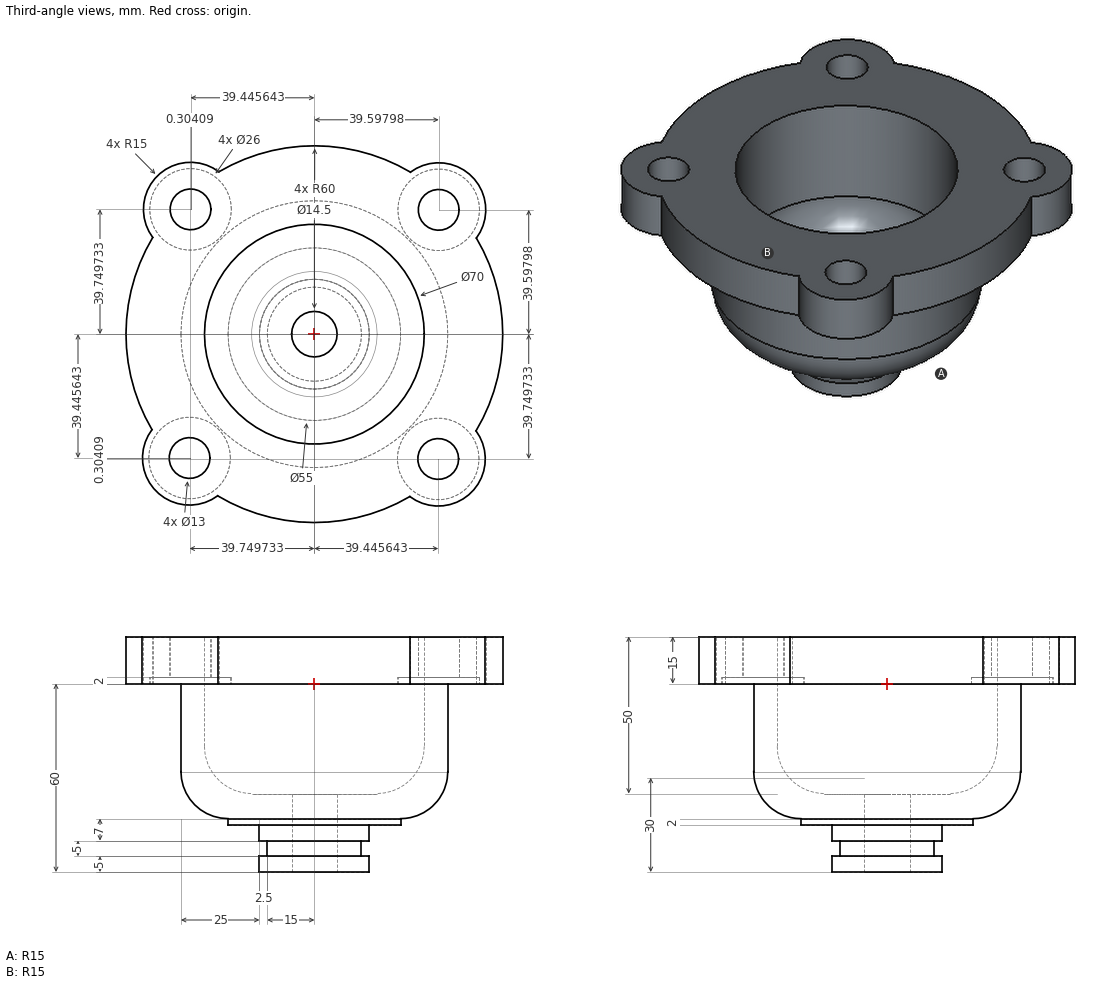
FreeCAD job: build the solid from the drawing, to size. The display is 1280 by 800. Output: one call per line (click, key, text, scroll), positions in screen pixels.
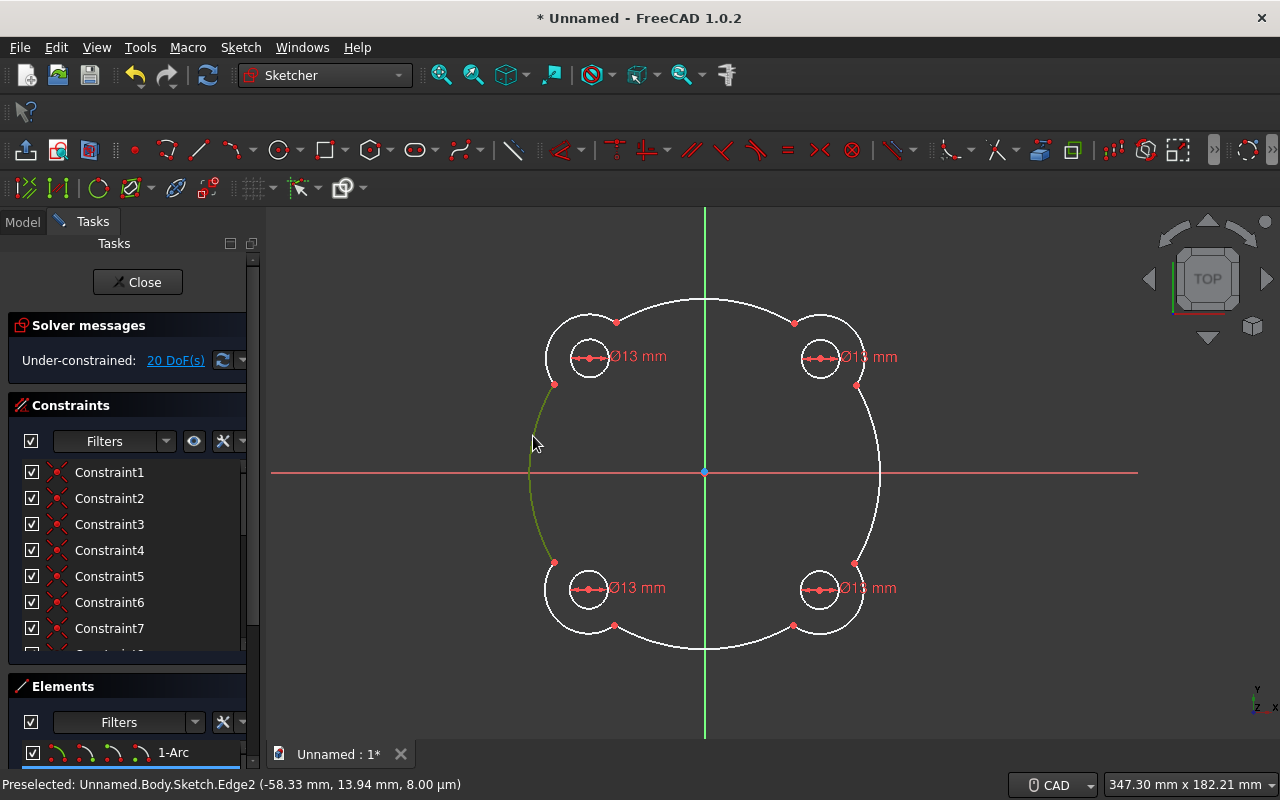
click(742, 303)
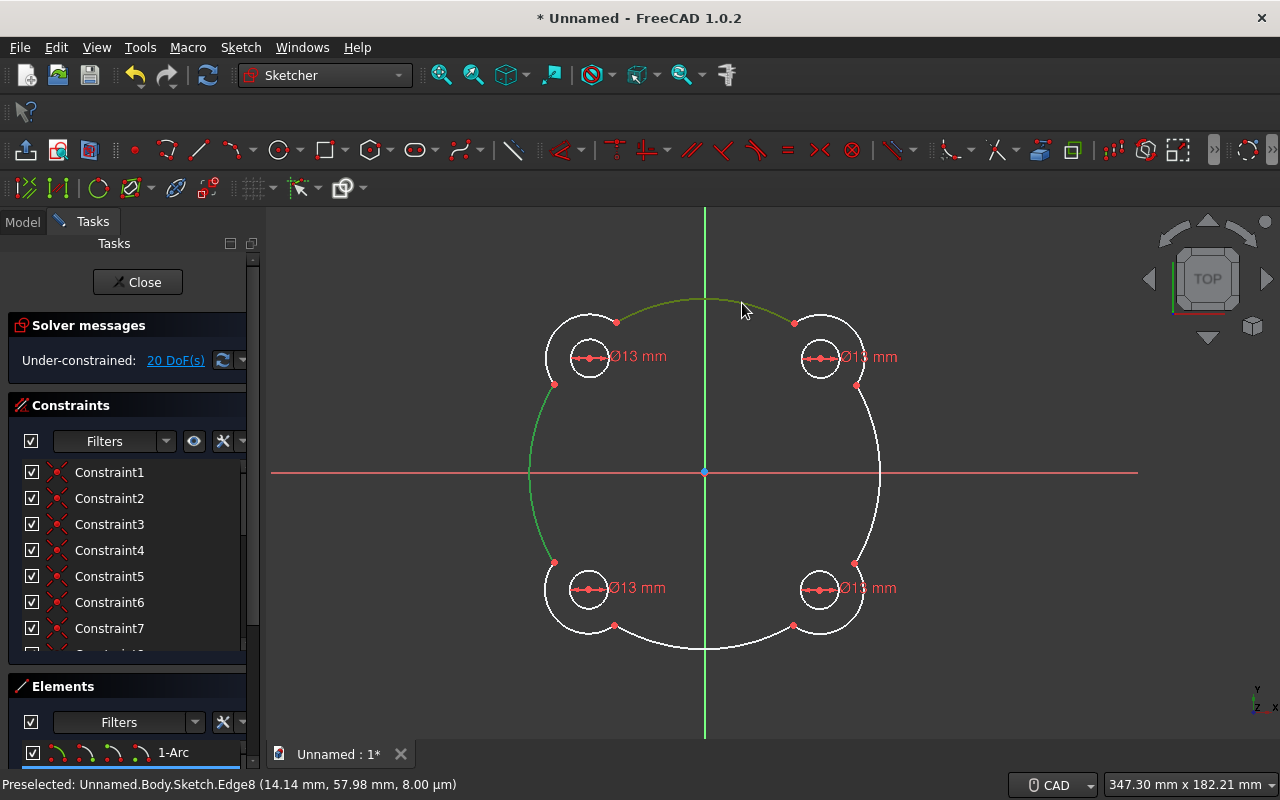
click(616, 150)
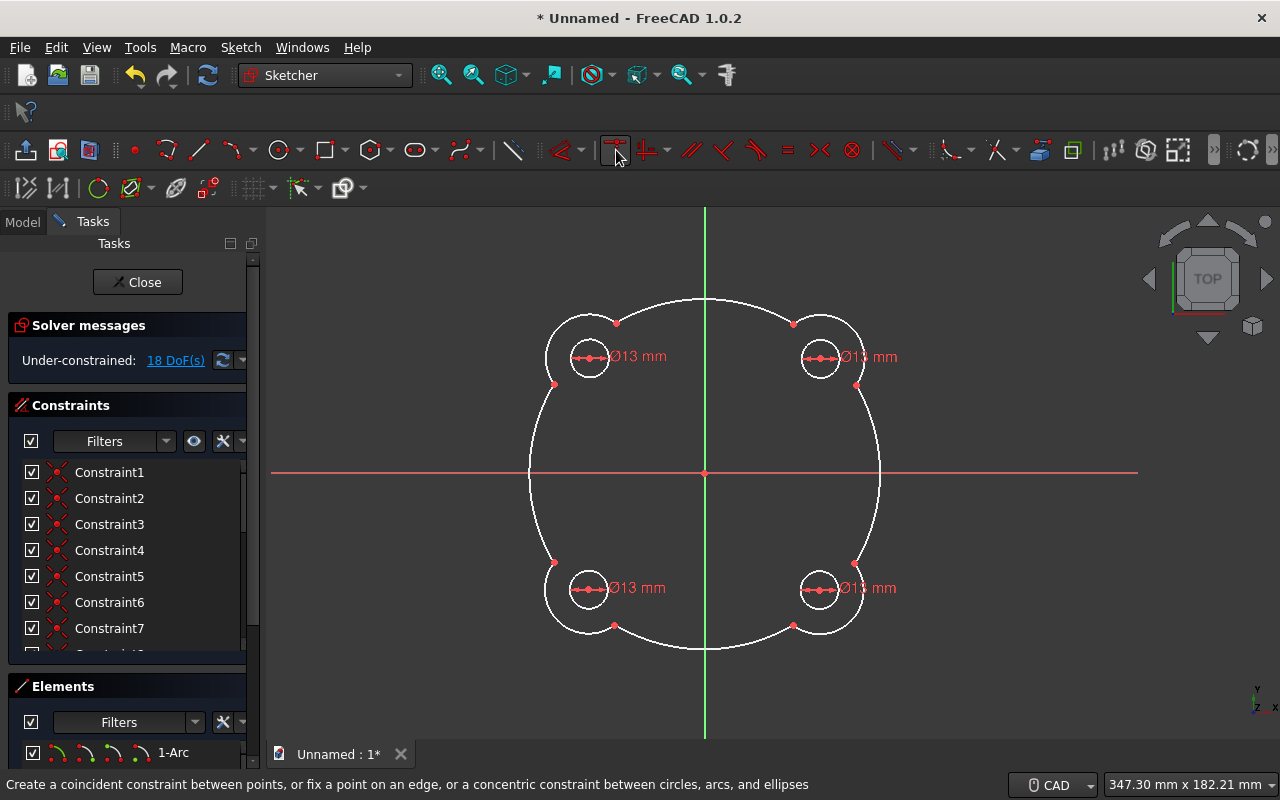
scroll(704, 473, up, 4)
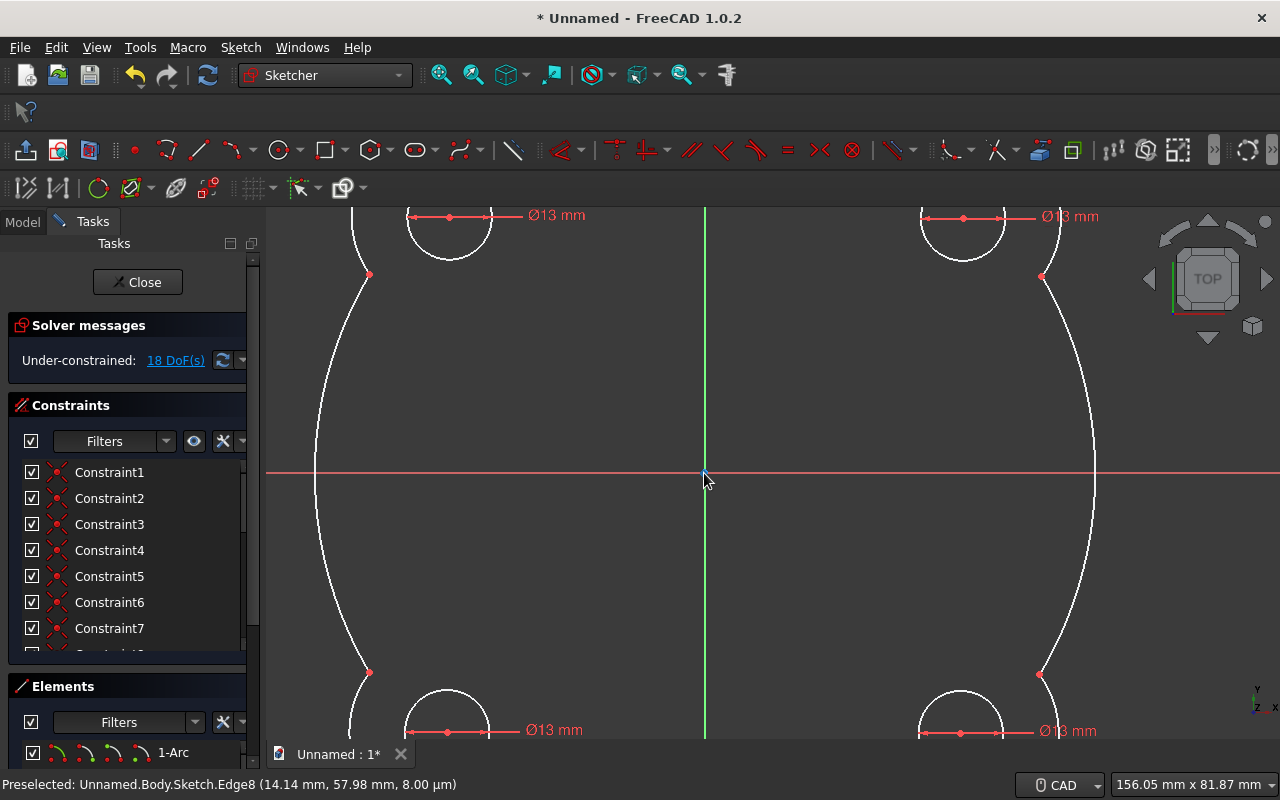
drag(694, 463, 715, 484)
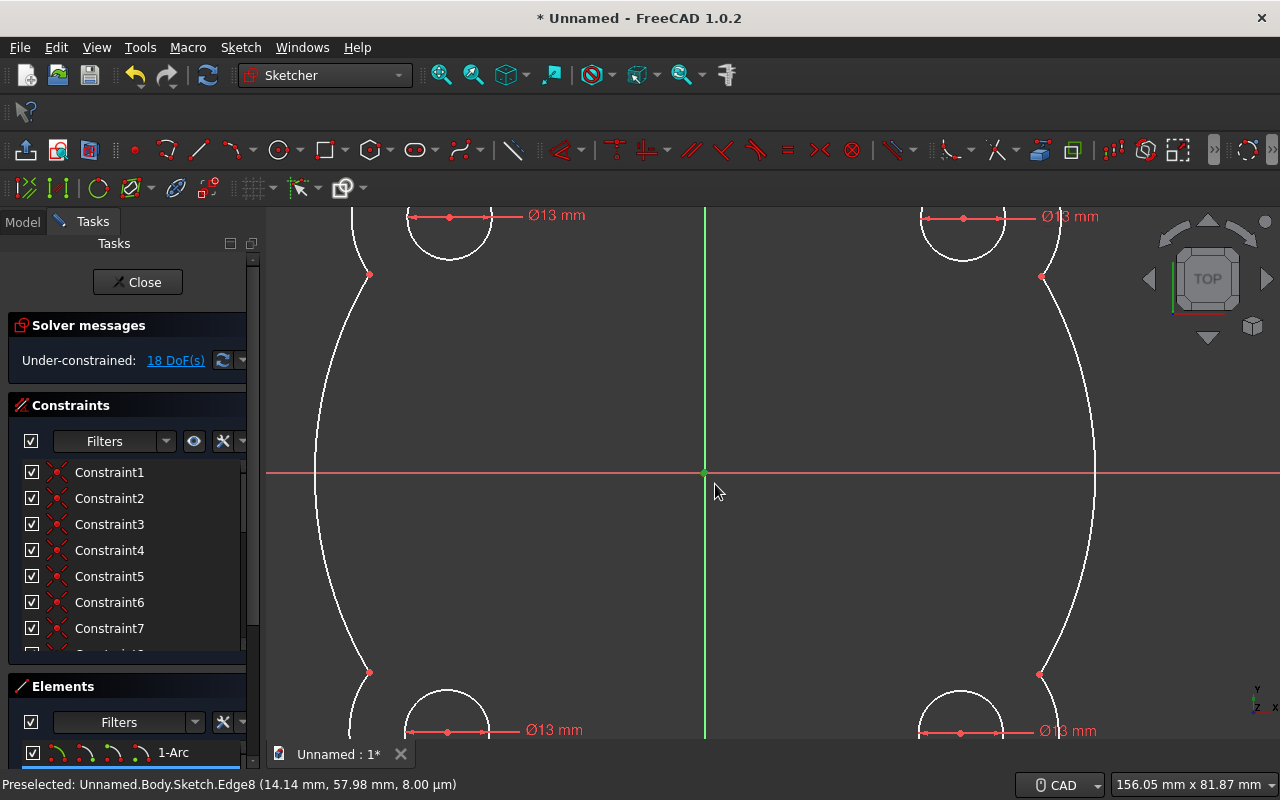
click(616, 150)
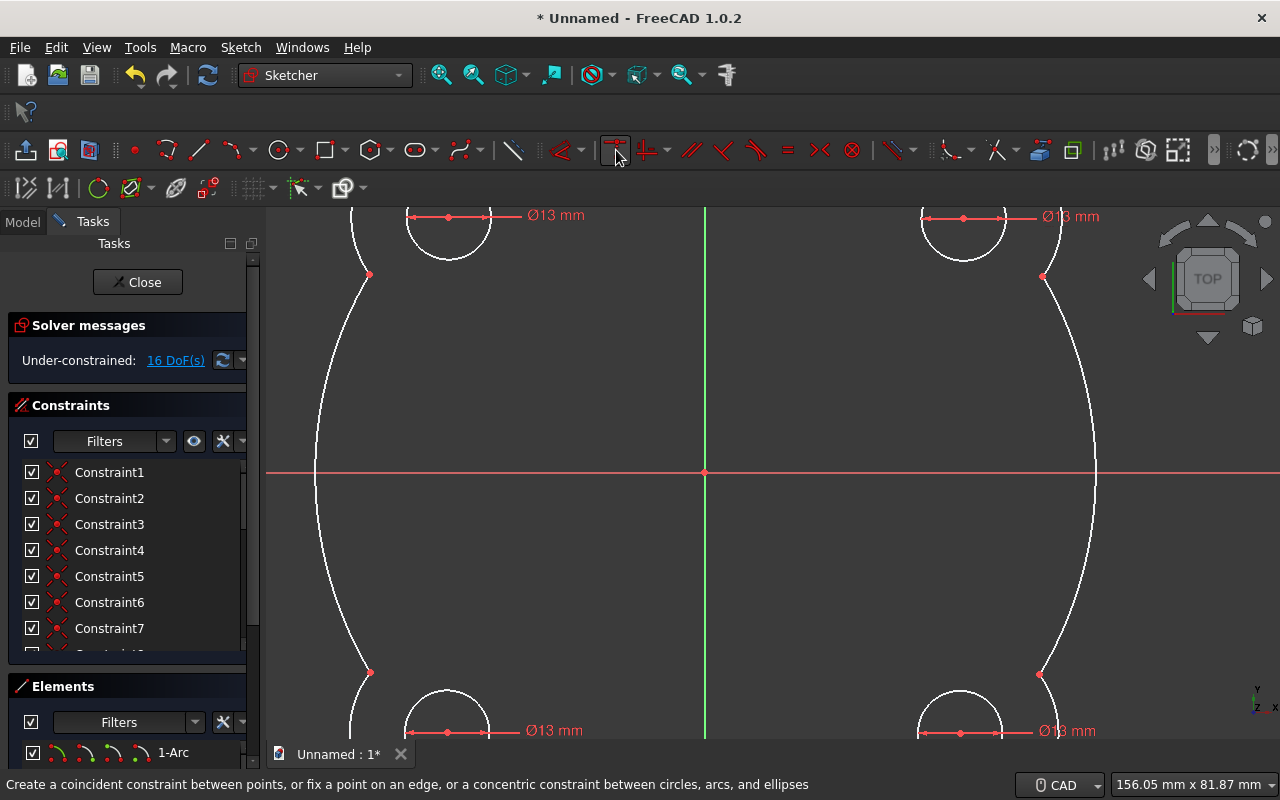
scroll(704, 473, down, 4)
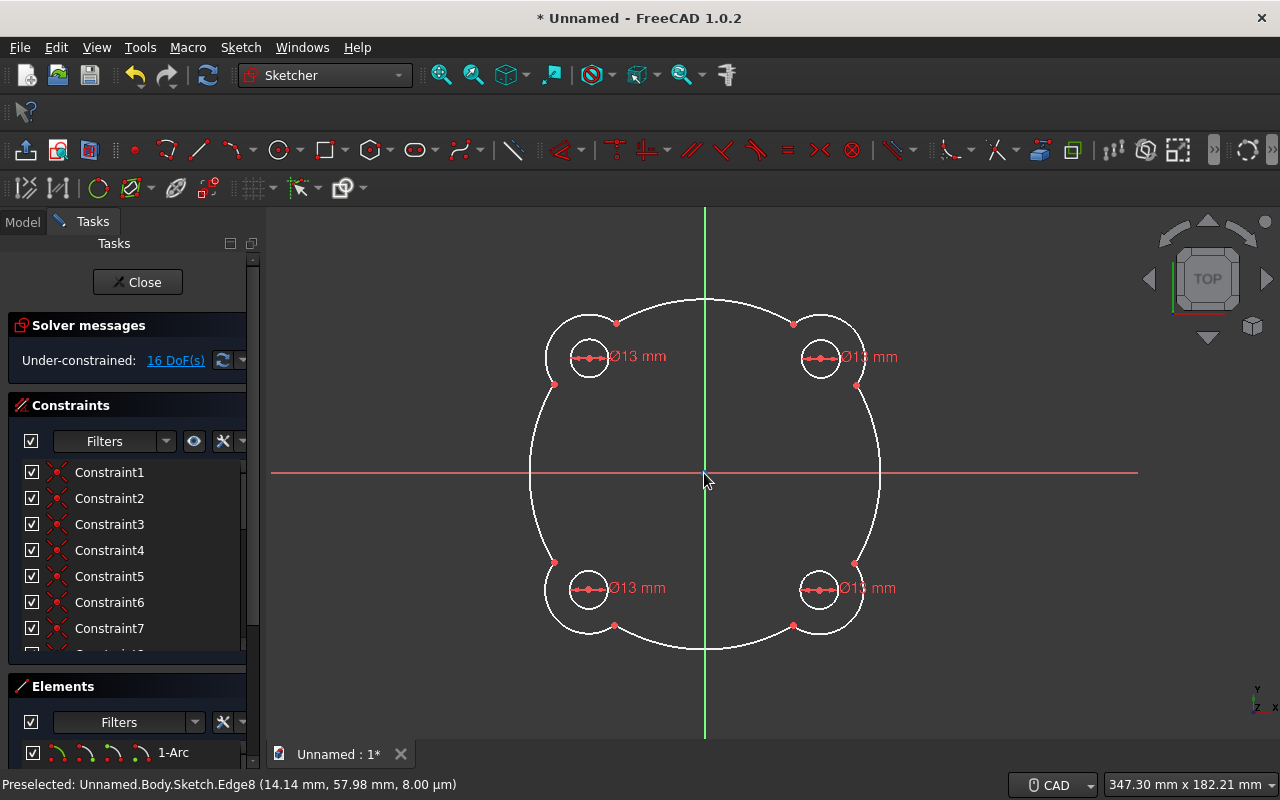
click(581, 316)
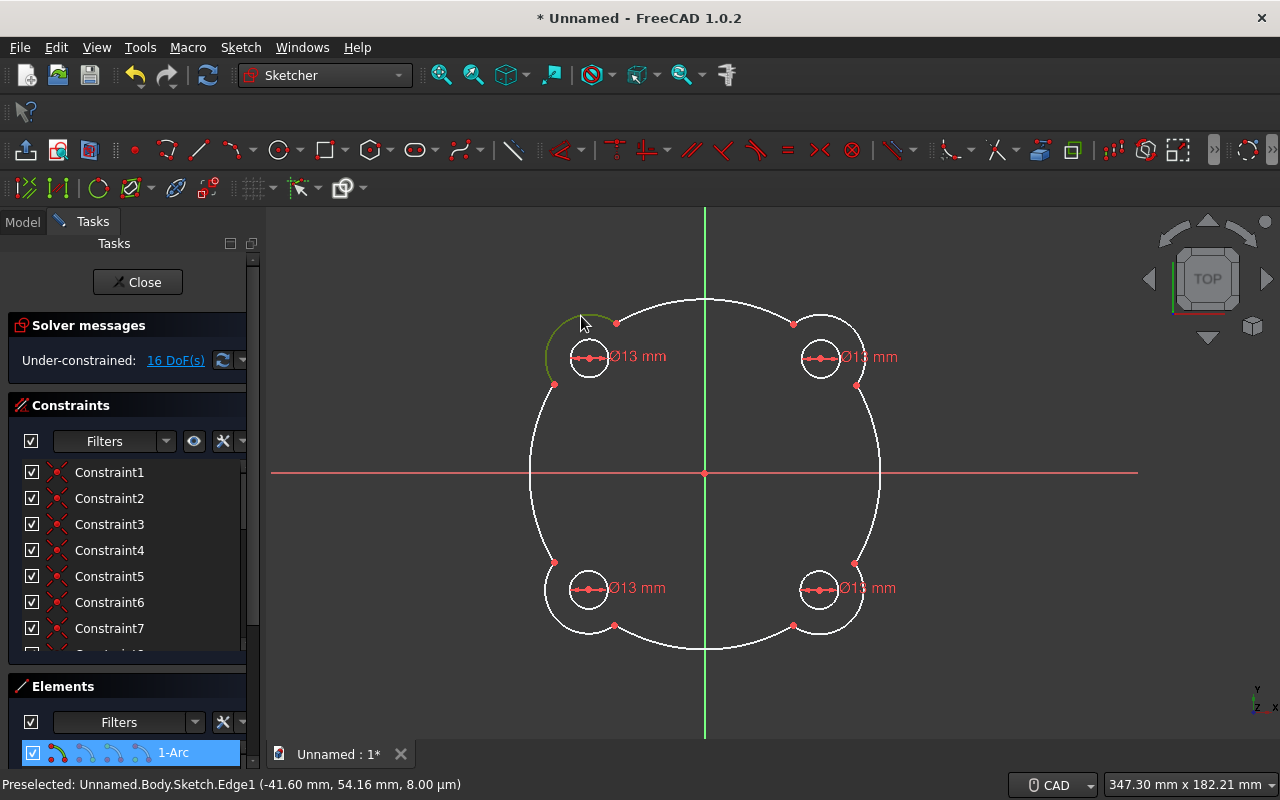
click(546, 599)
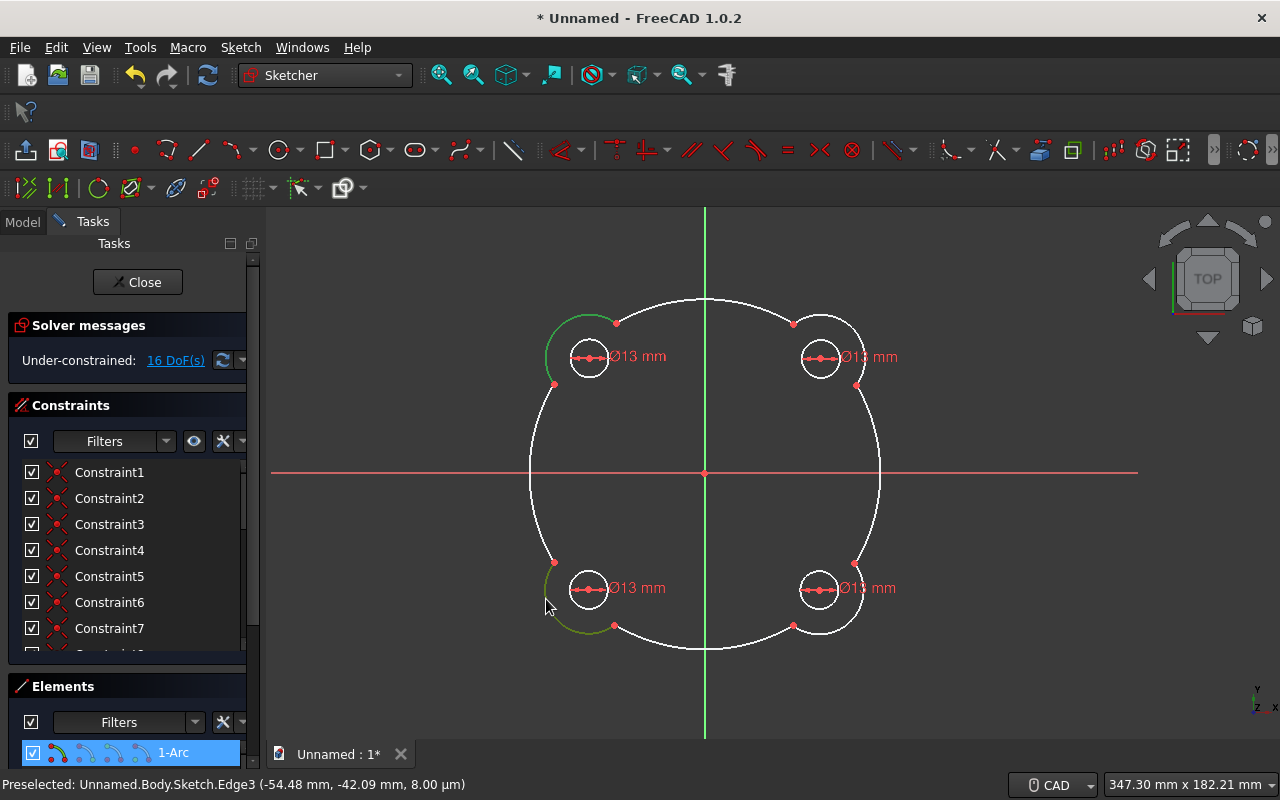
click(829, 633)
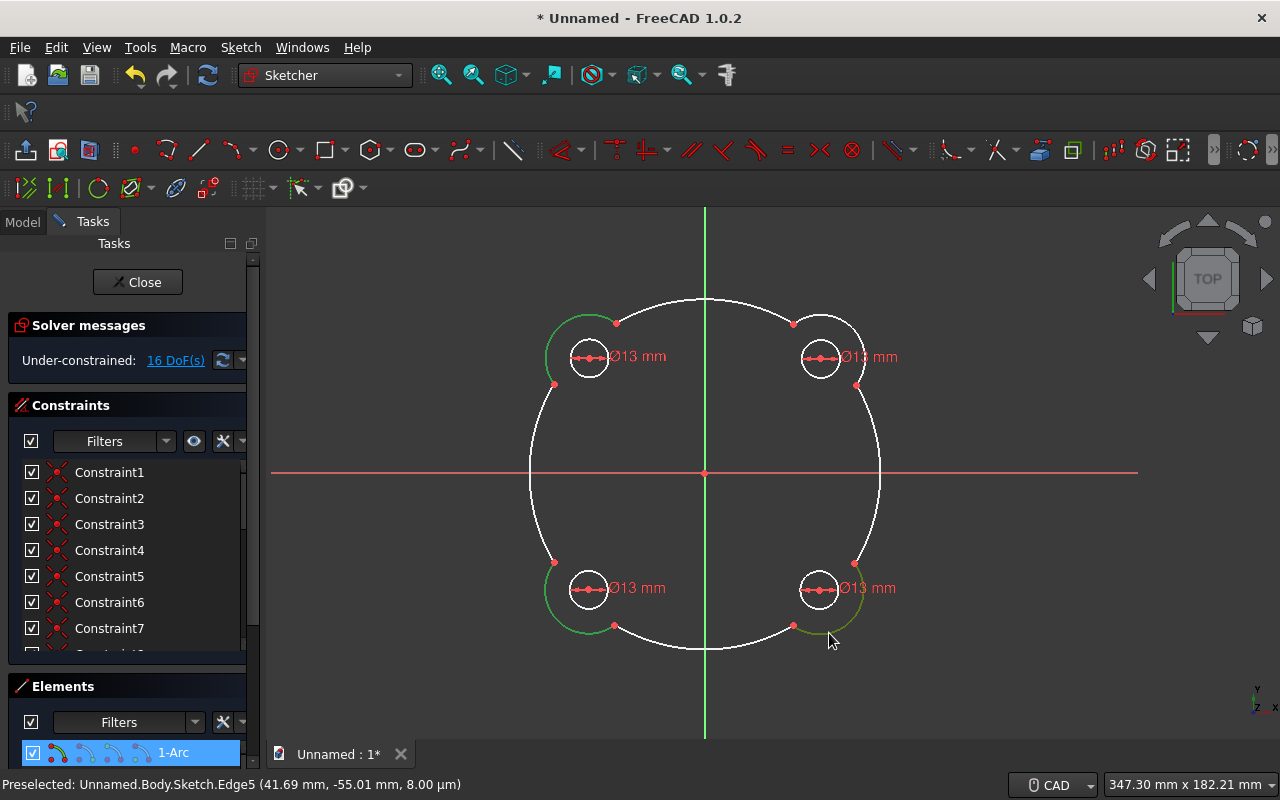
click(864, 349)